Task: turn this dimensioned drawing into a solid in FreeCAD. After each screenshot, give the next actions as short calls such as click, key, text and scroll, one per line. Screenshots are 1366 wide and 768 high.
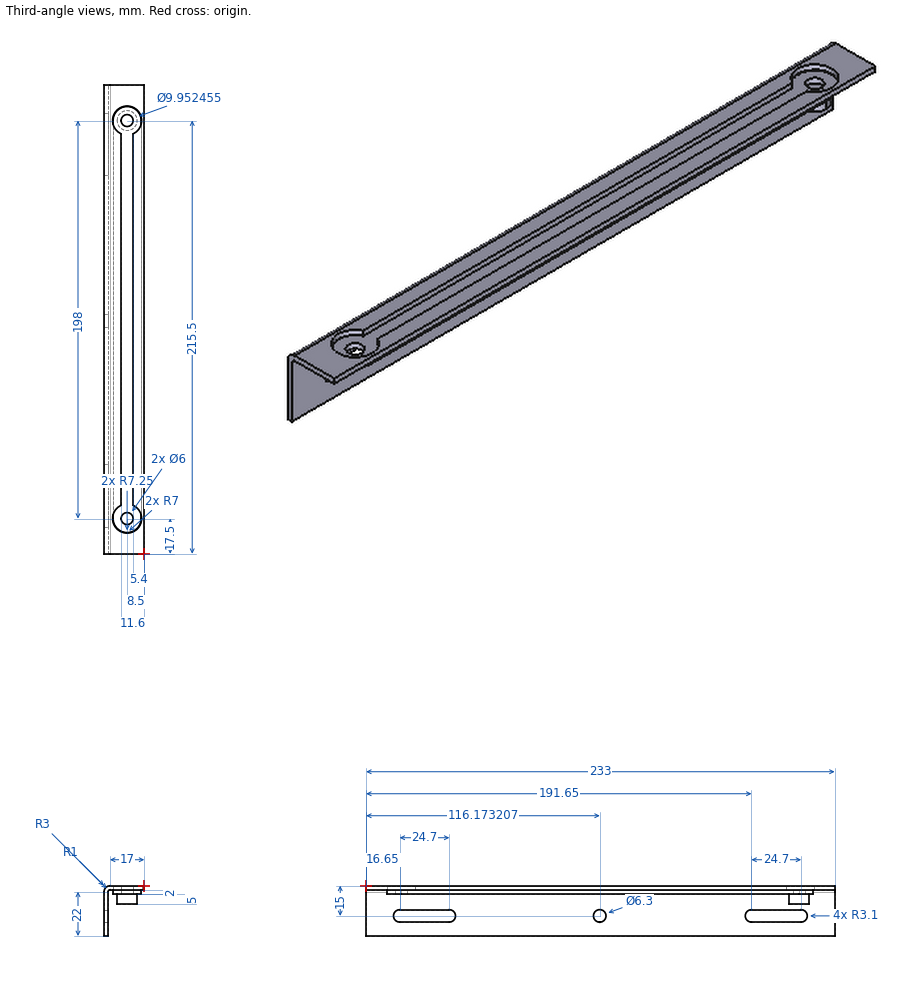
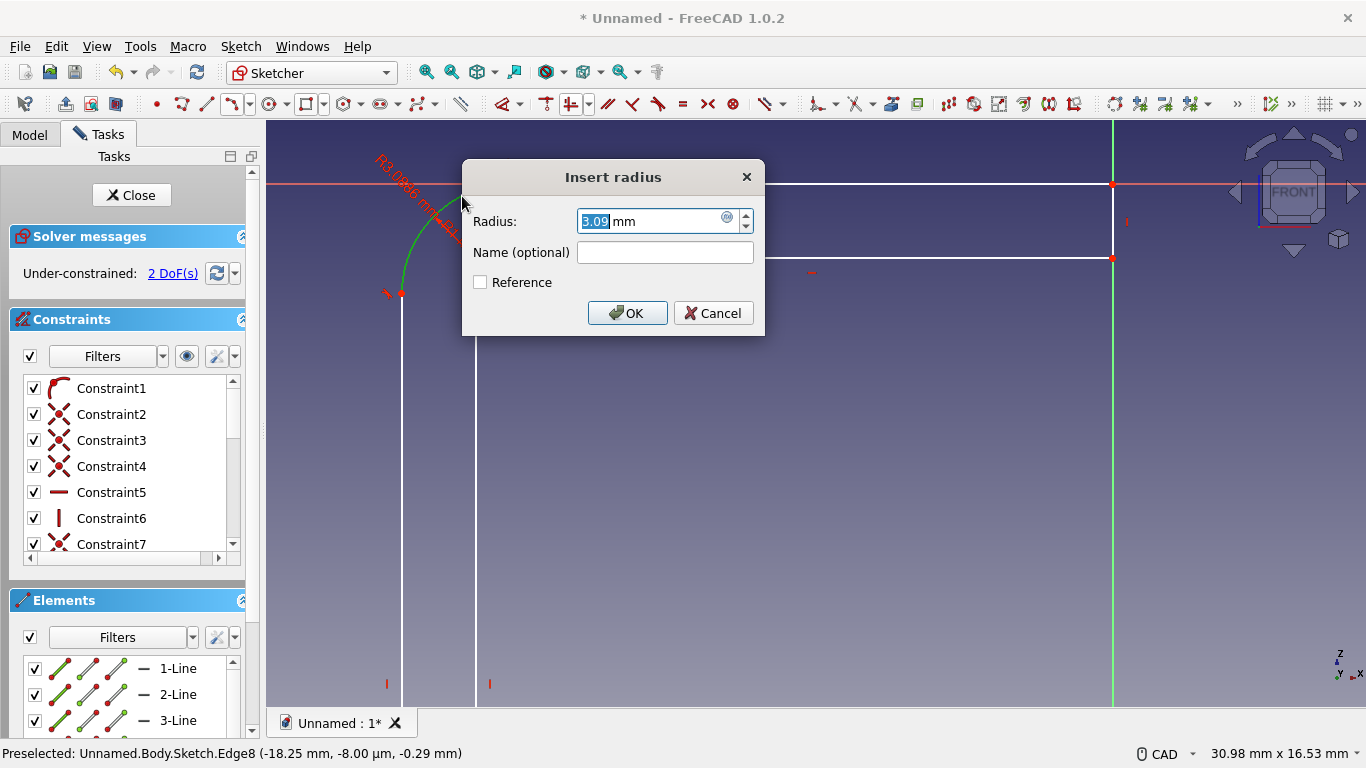
text(3)
key(Return)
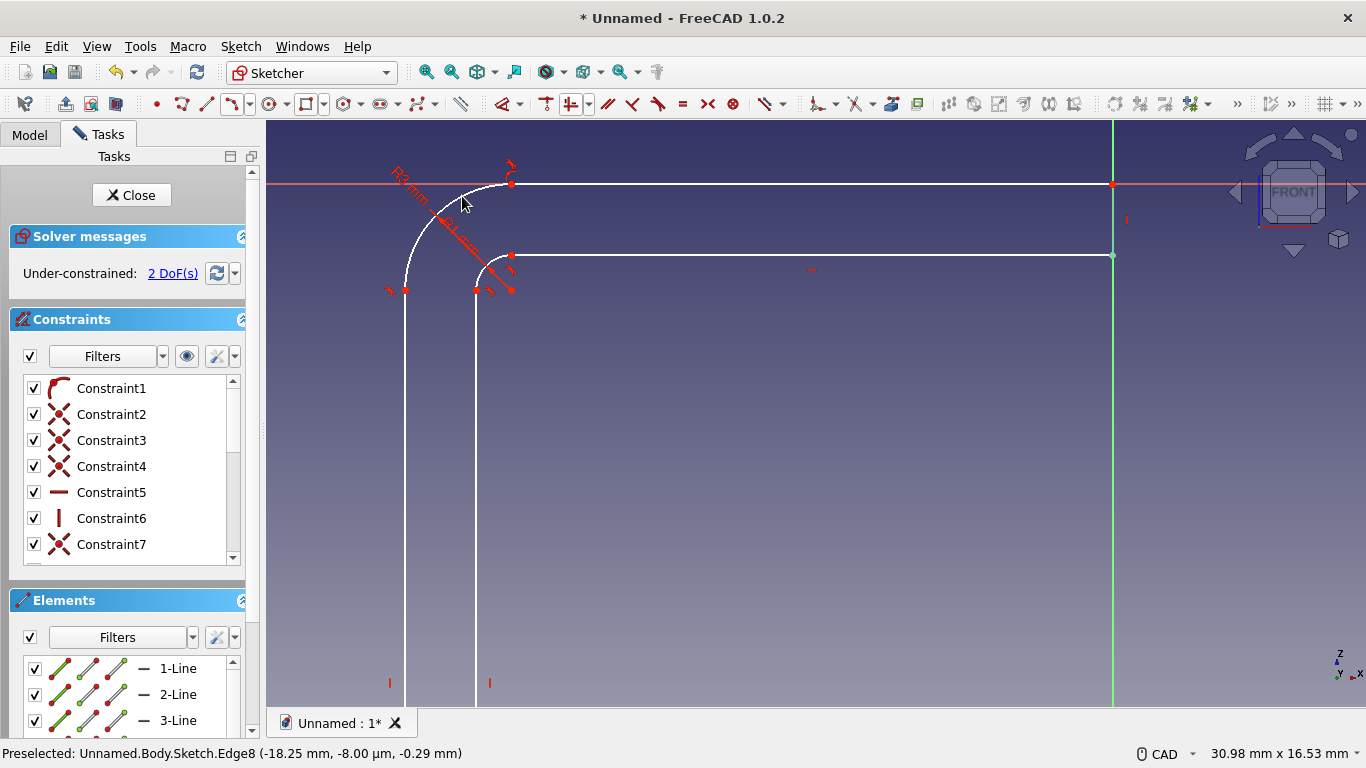
click(692, 184)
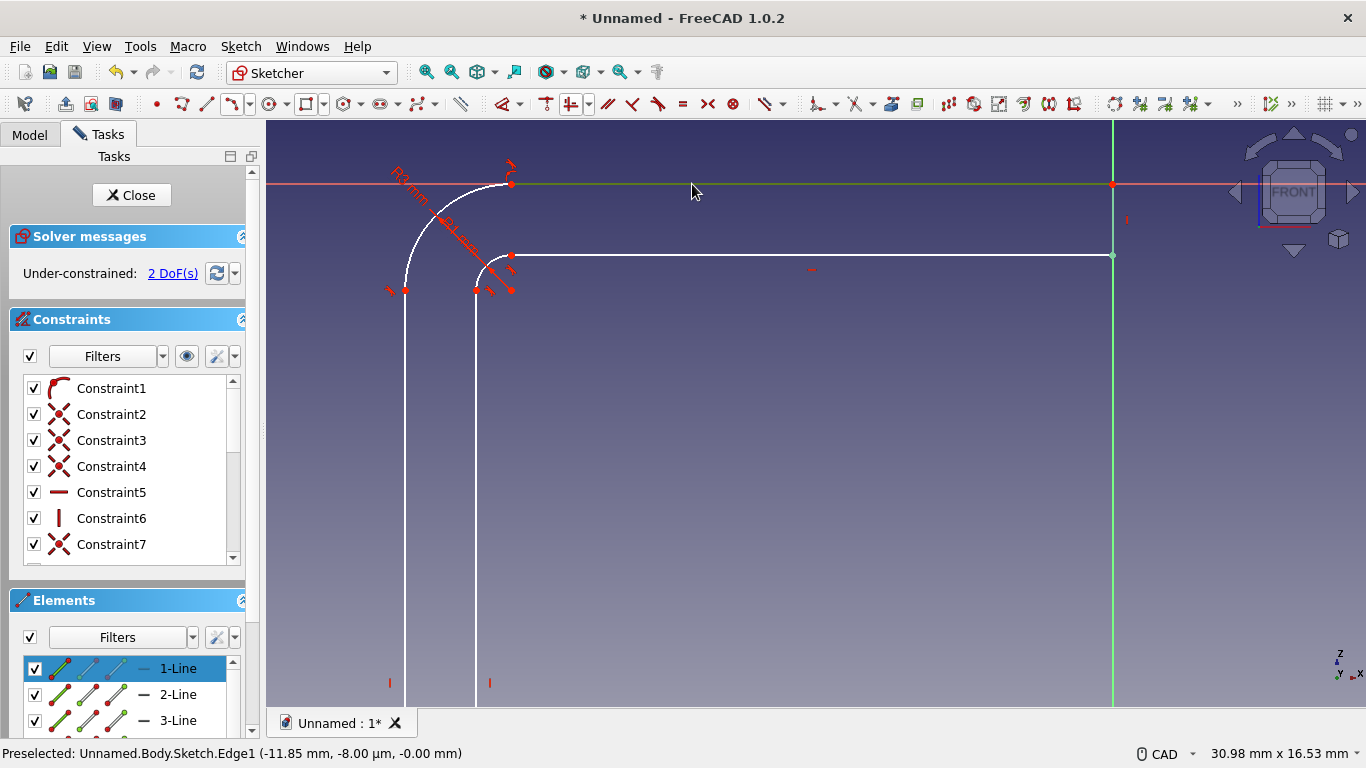
key(l)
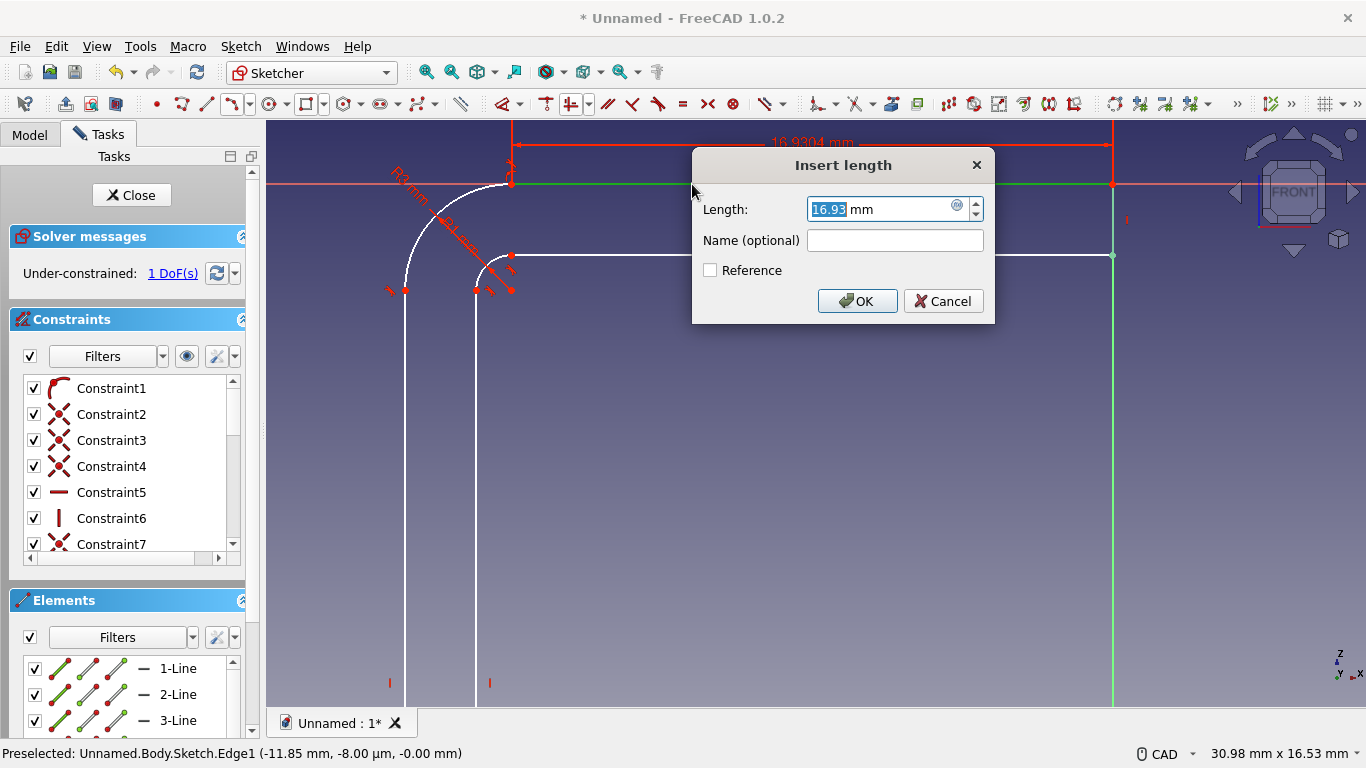
text(17)
key(Return)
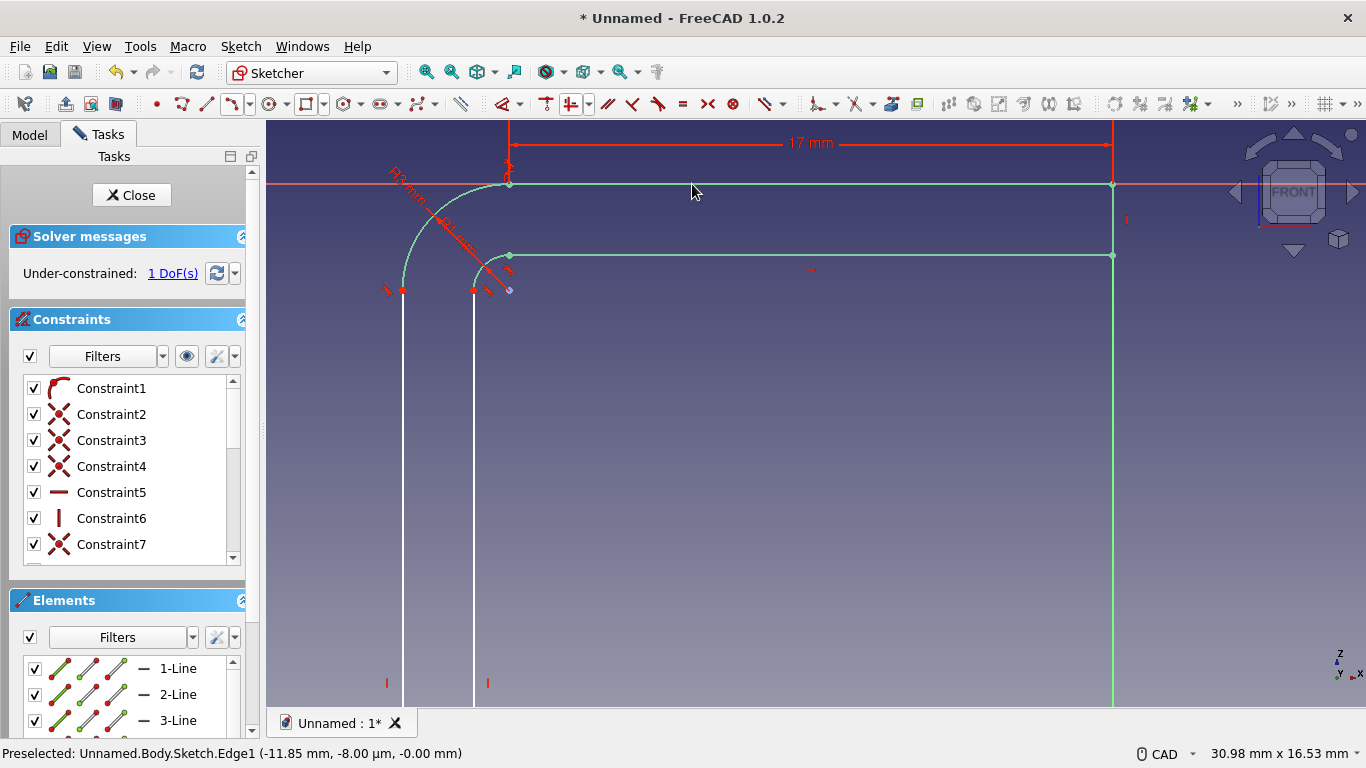
click(474, 526)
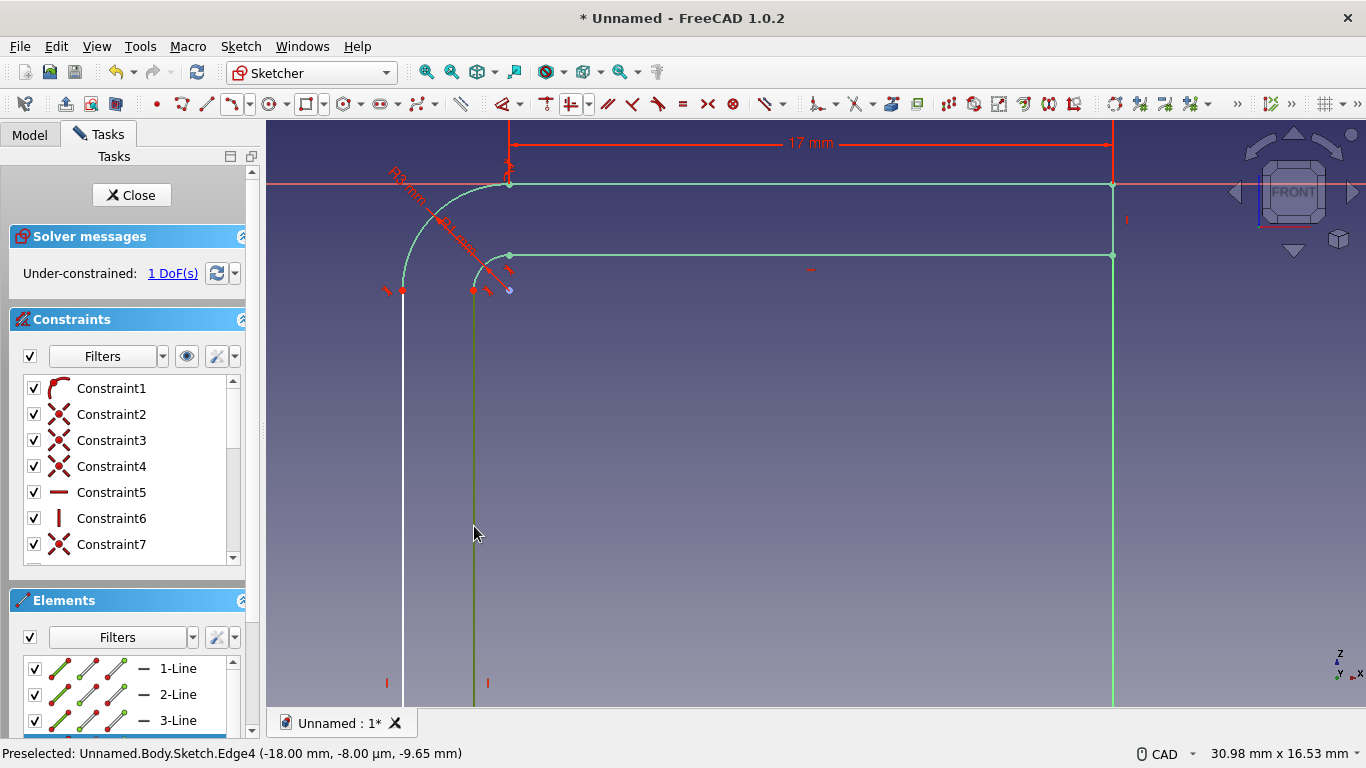
click(520, 104)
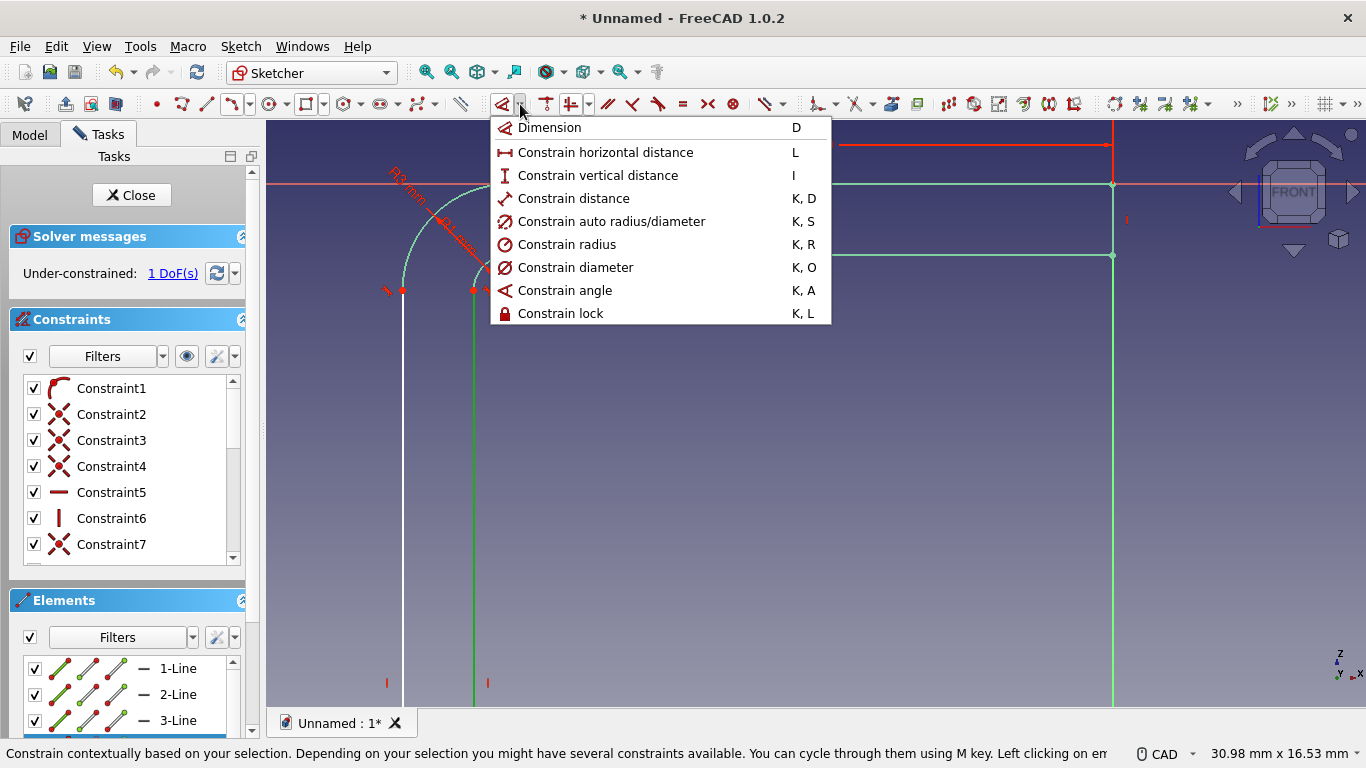
click(661, 176)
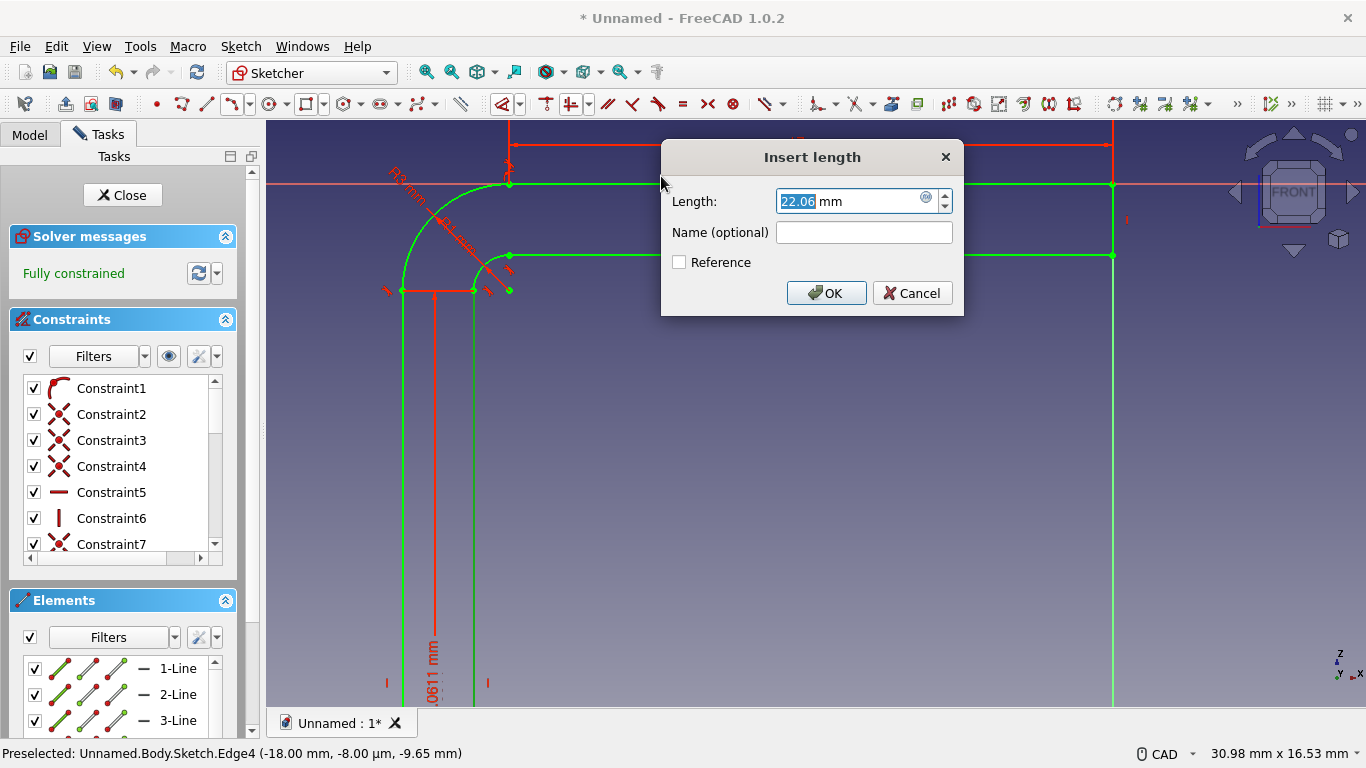
text(22)
key(Return)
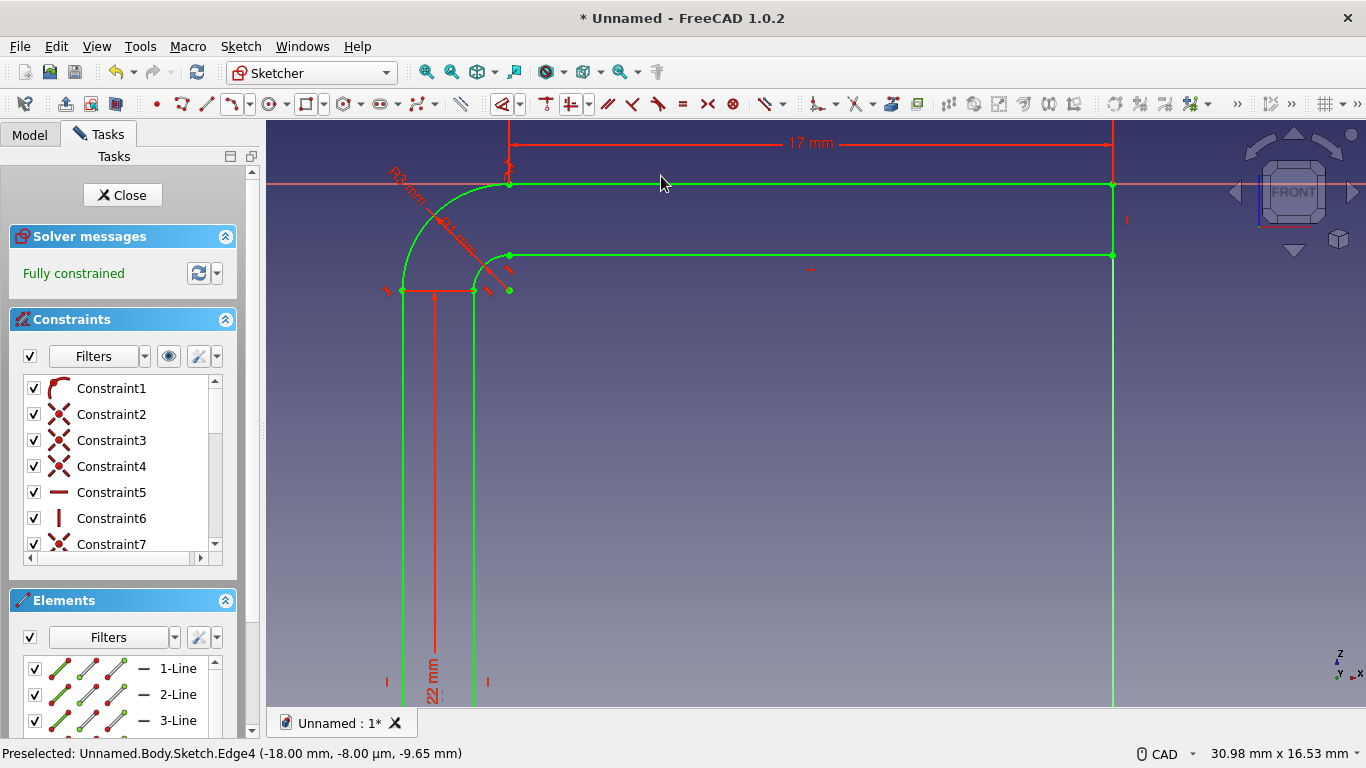
click(123, 195)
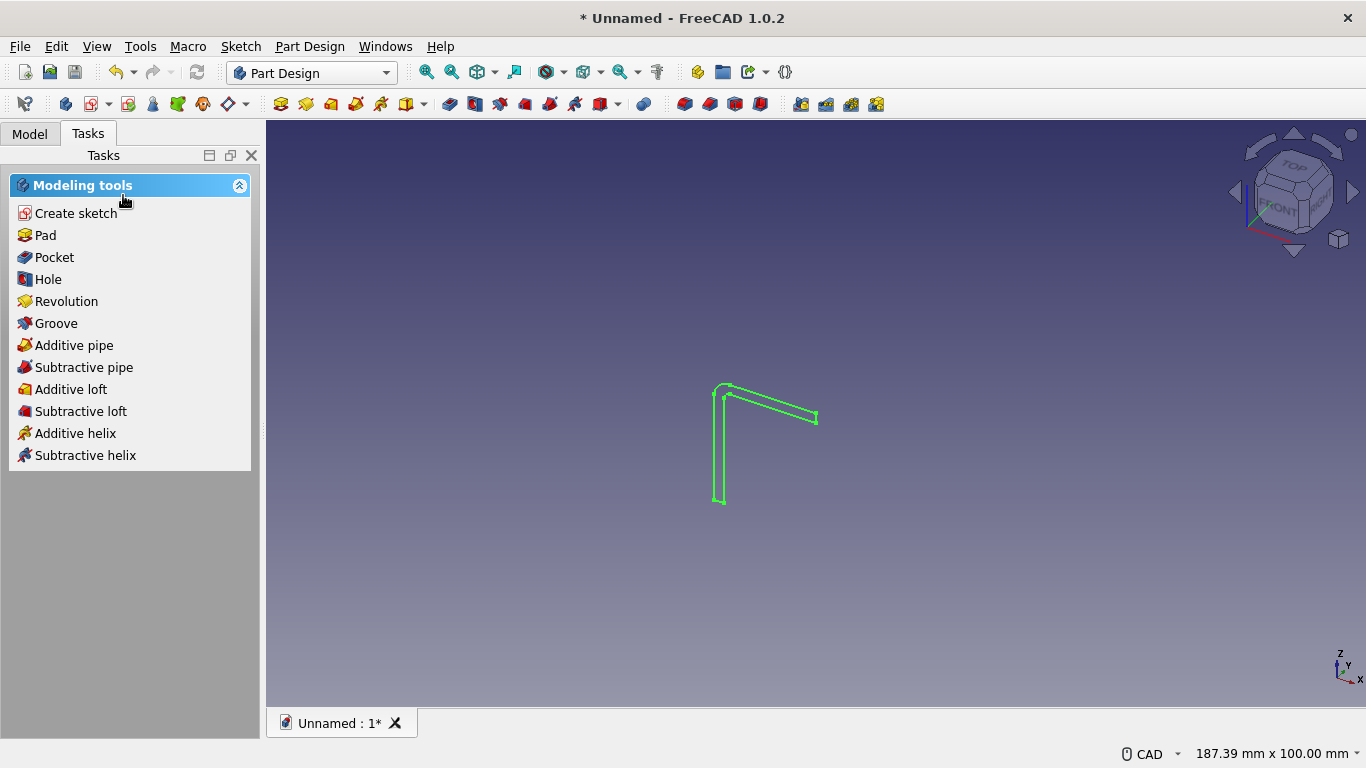
click(281, 104)